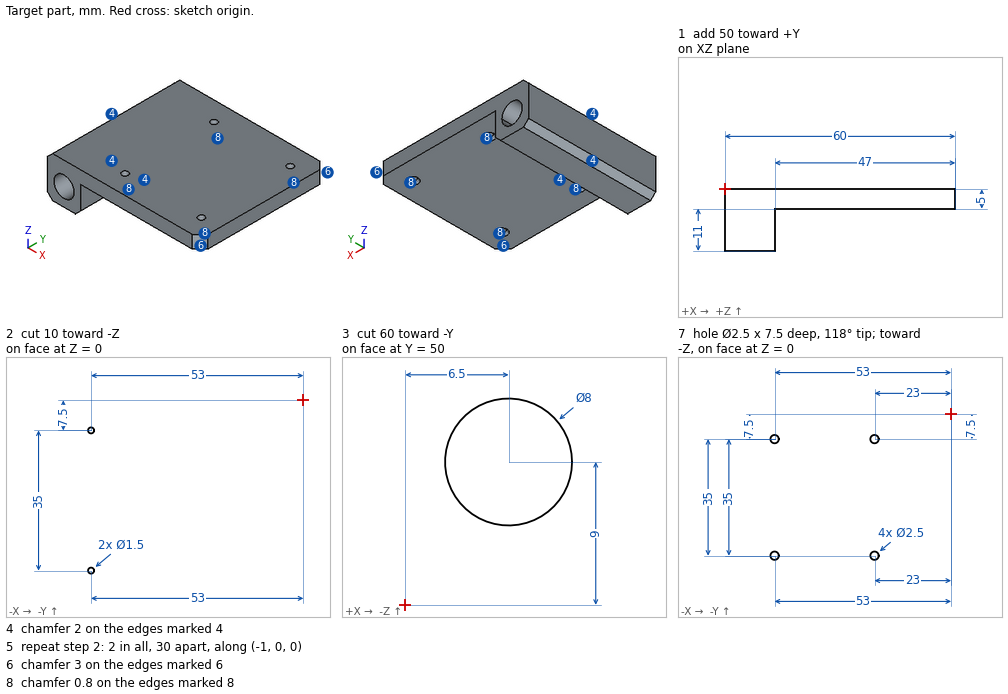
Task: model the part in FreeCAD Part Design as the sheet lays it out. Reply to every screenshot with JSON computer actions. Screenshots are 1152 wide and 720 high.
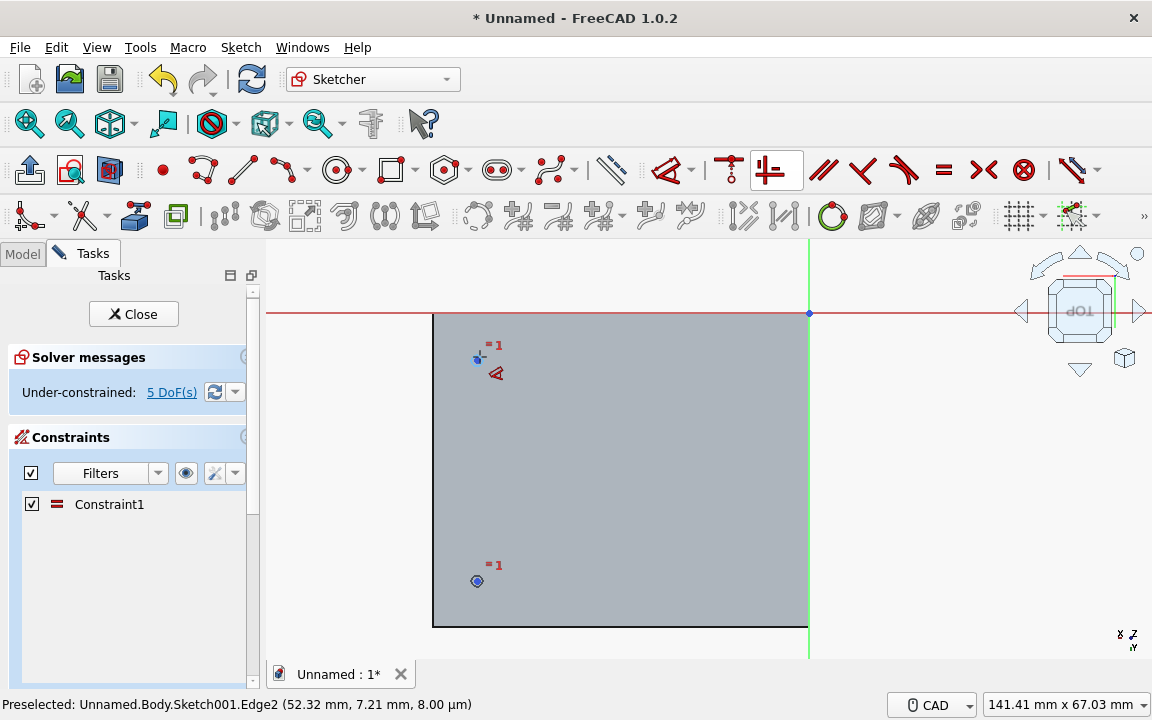
{"action": "scroll", "coordinate": [481, 577], "scroll_direction": "up", "scroll_amount": 8}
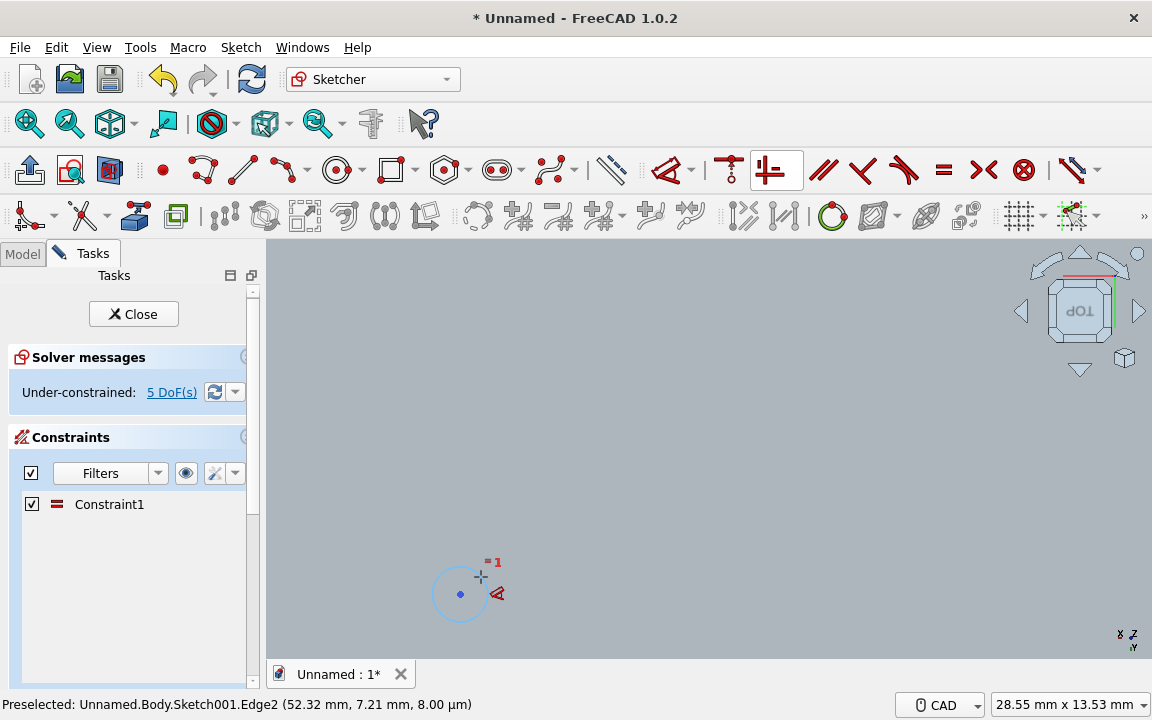
{"action": "left_click", "coordinate": [480, 575]}
{"action": "left_click", "coordinate": [503, 553]}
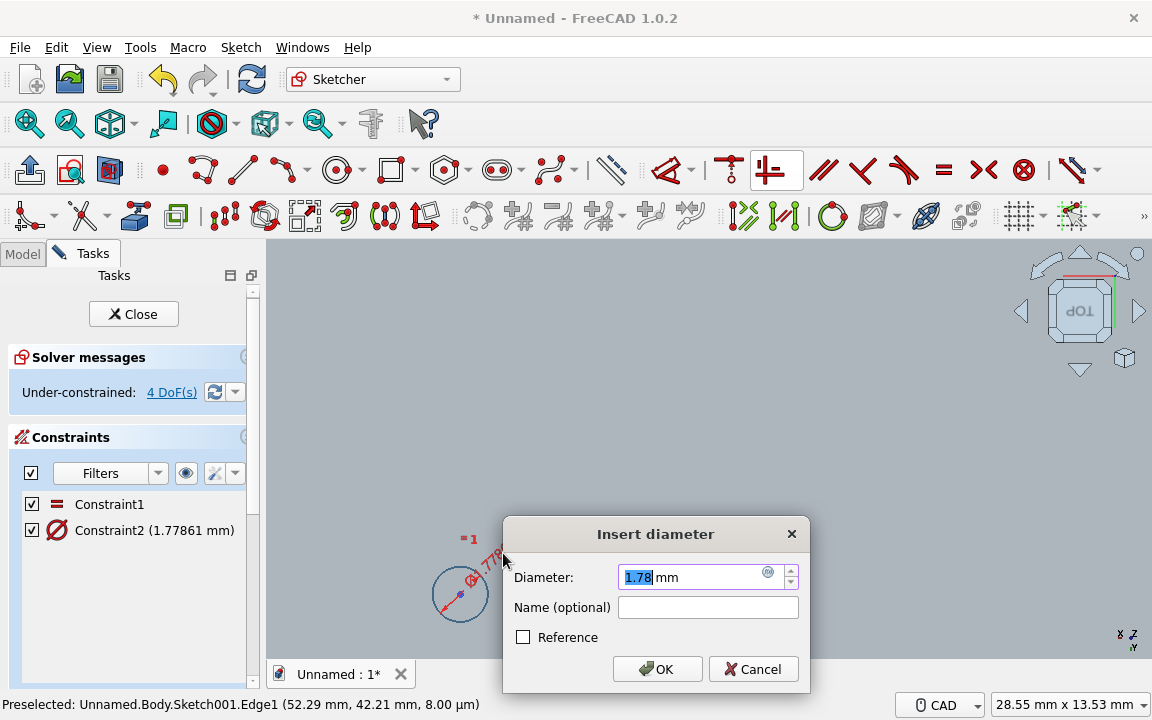
{"action": "type", "text": "1.5"}
{"action": "key", "text": "Return"}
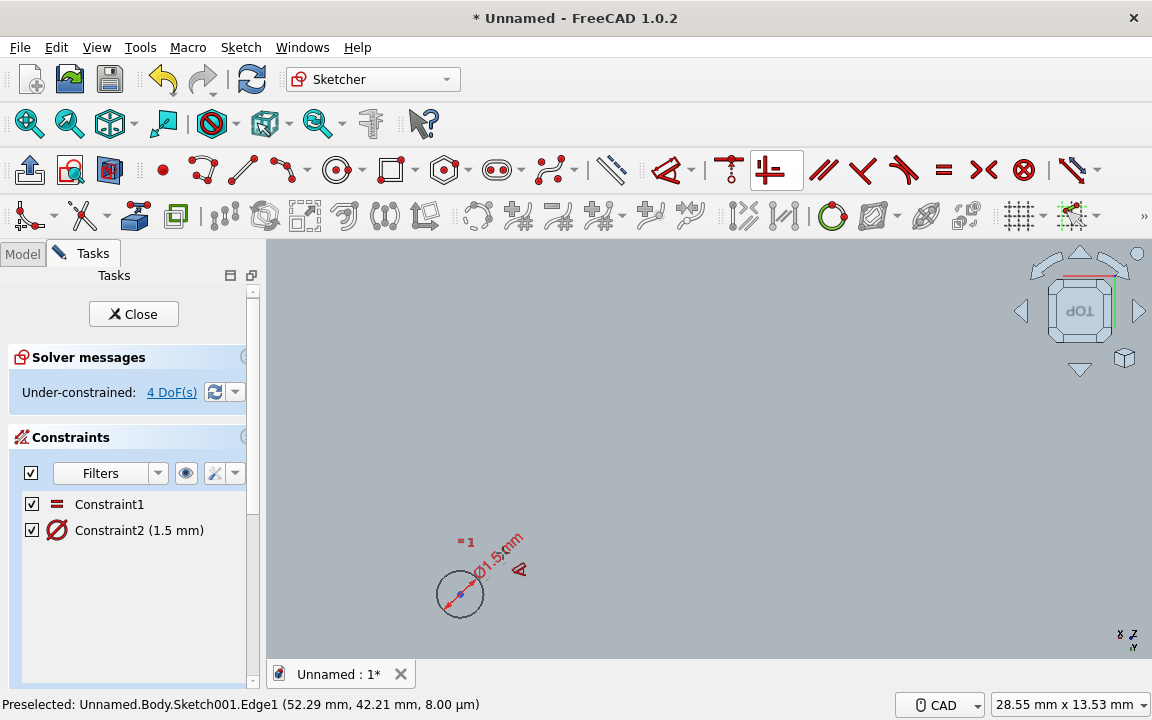
{"action": "scroll", "coordinate": [481, 578], "scroll_direction": "down", "scroll_amount": 8}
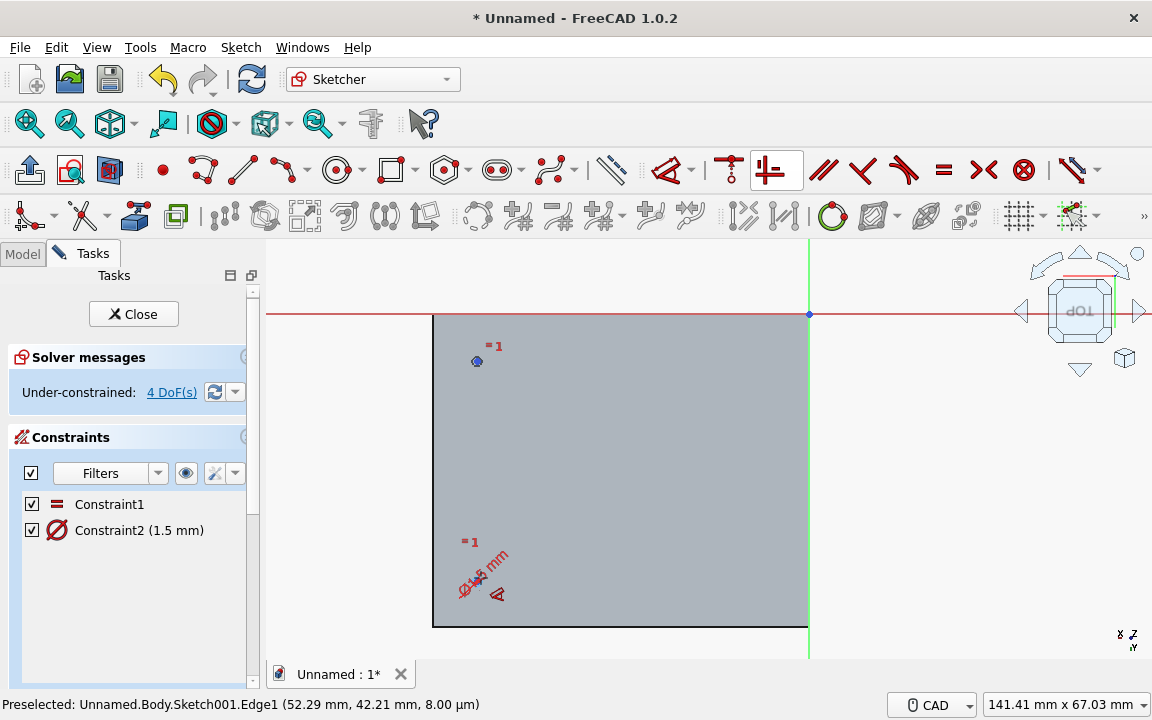
{"action": "left_click", "coordinate": [477, 582]}
{"action": "left_click", "coordinate": [643, 280]}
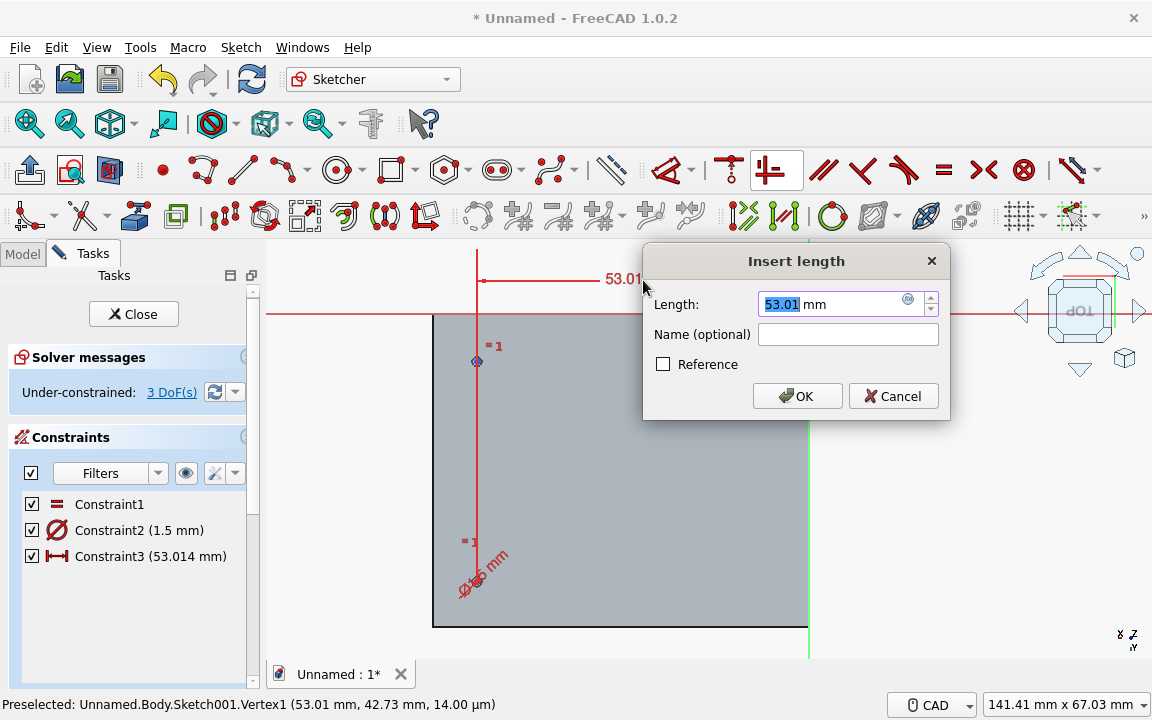
{"action": "type", "text": "53"}
{"action": "key", "text": "Return"}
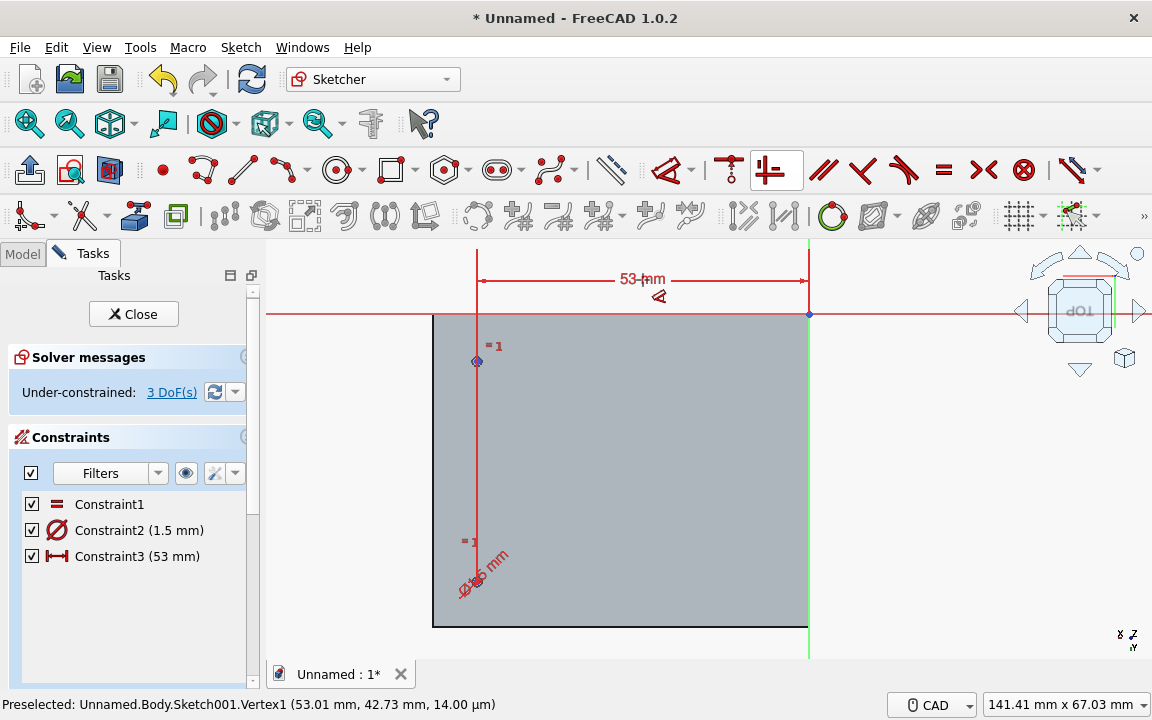
{"action": "left_click", "coordinate": [477, 362]}
{"action": "left_click", "coordinate": [567, 280]}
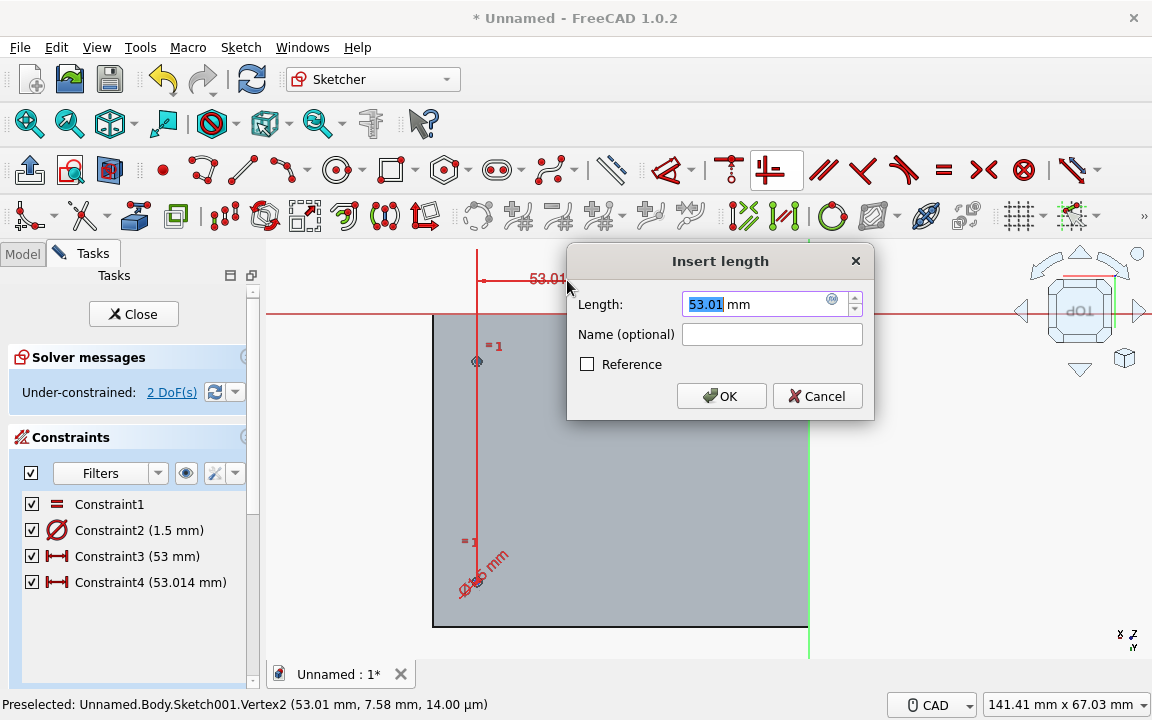
{"action": "type", "text": "53"}
{"action": "key", "text": "Return"}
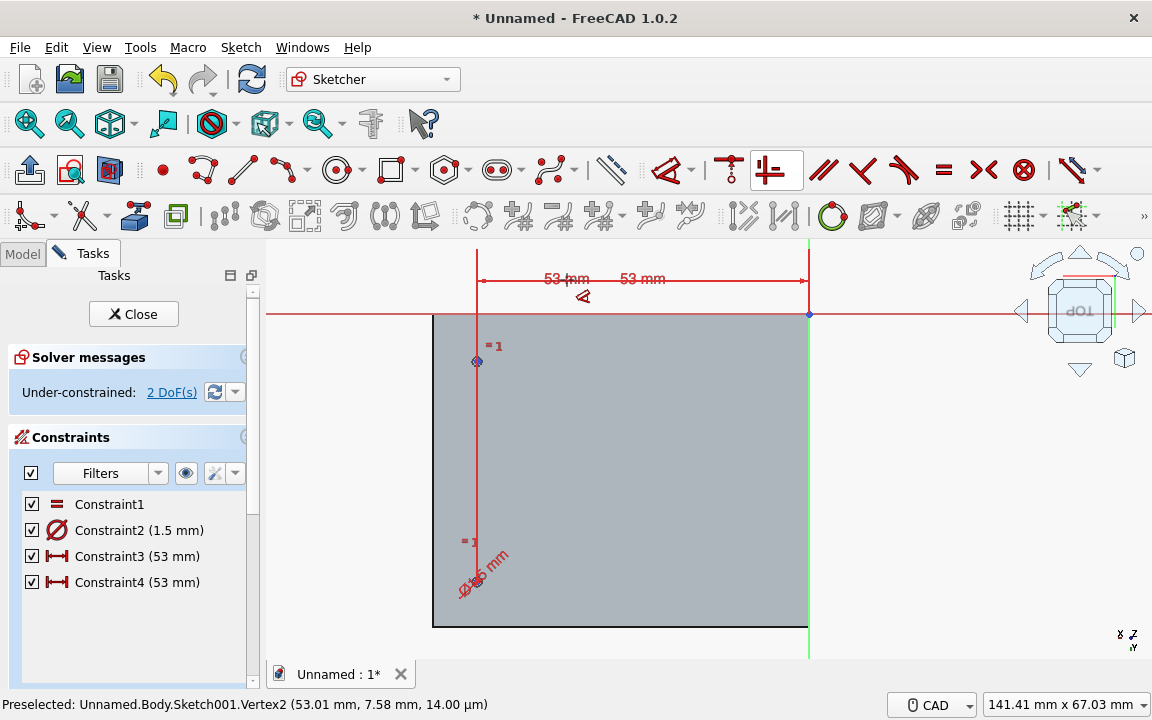
{"action": "left_click", "coordinate": [477, 362]}
{"action": "left_click", "coordinate": [843, 338]}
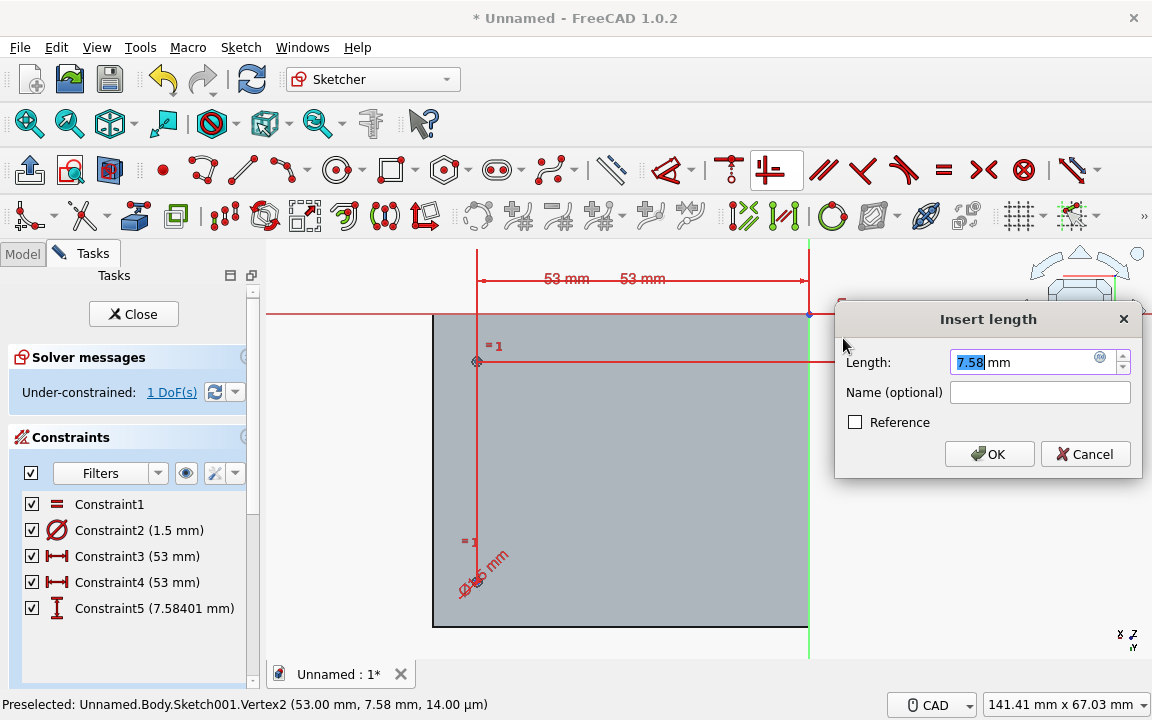
{"action": "type", "text": "7.5"}
{"action": "key", "text": "Return"}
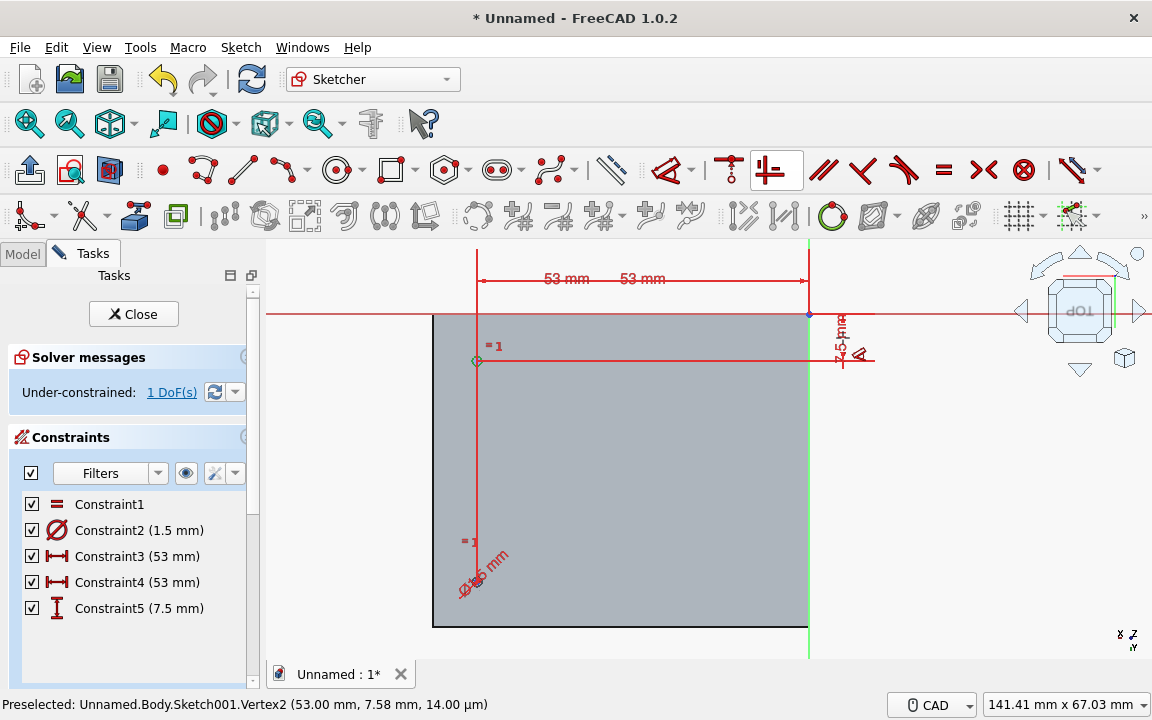
{"action": "left_click", "coordinate": [477, 582]}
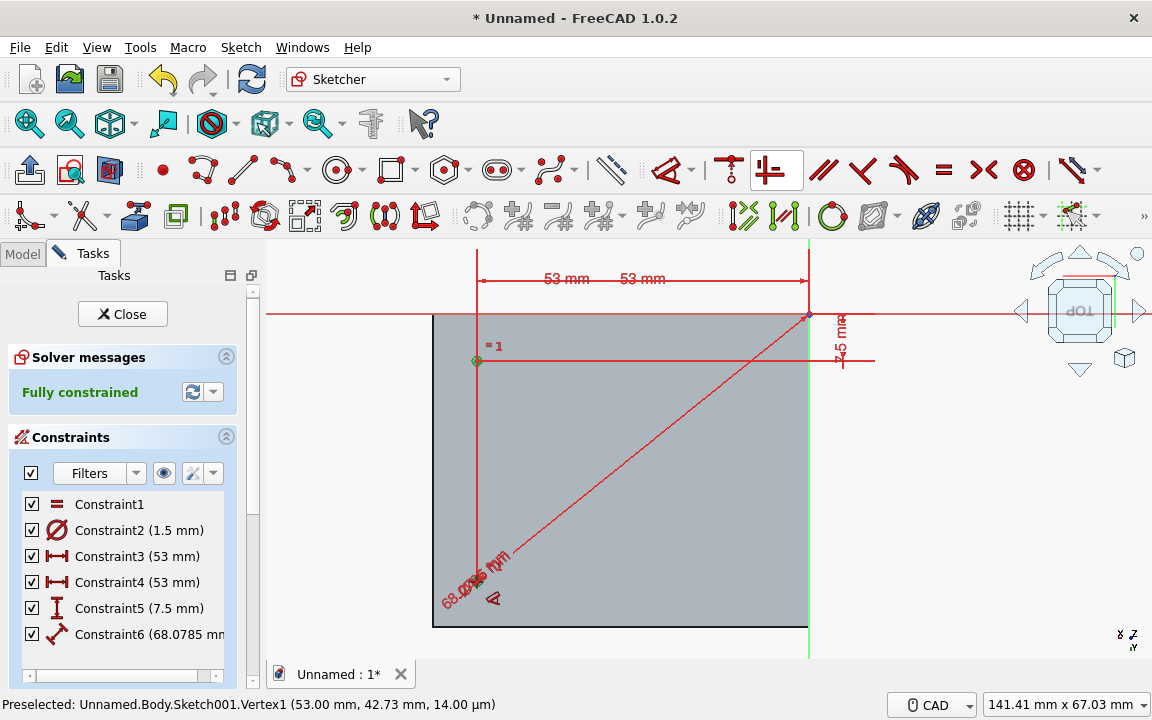
{"action": "left_click", "coordinate": [477, 361]}
{"action": "left_click", "coordinate": [443, 472]}